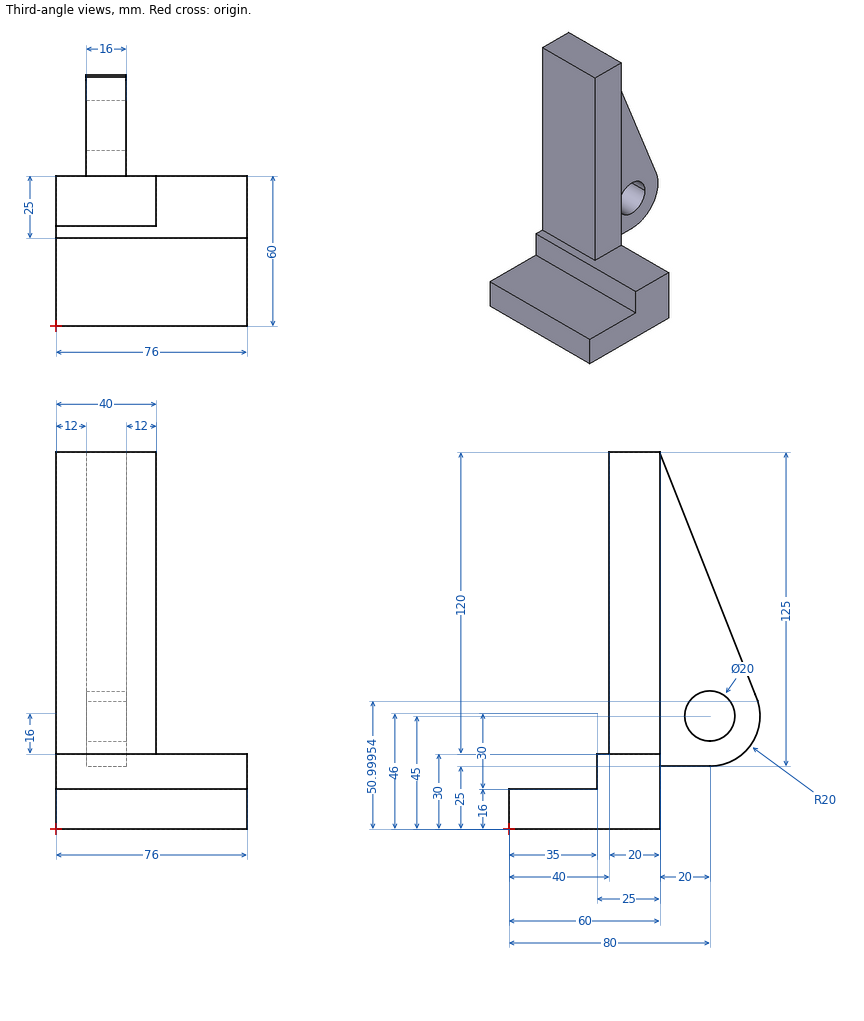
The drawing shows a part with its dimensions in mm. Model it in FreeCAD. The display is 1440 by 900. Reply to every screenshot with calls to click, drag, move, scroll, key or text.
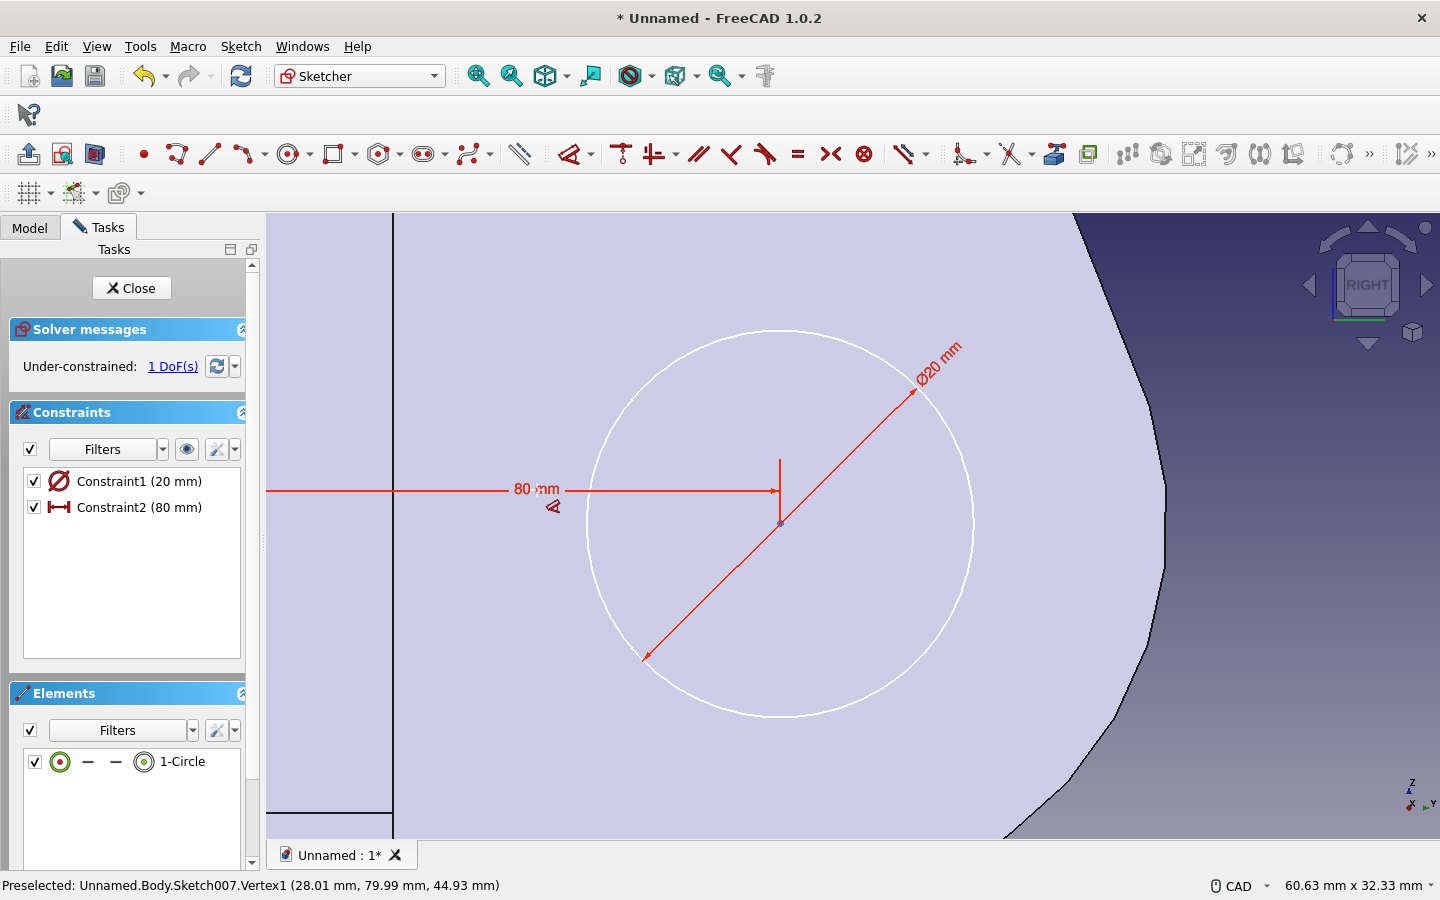
click(780, 524)
click(814, 668)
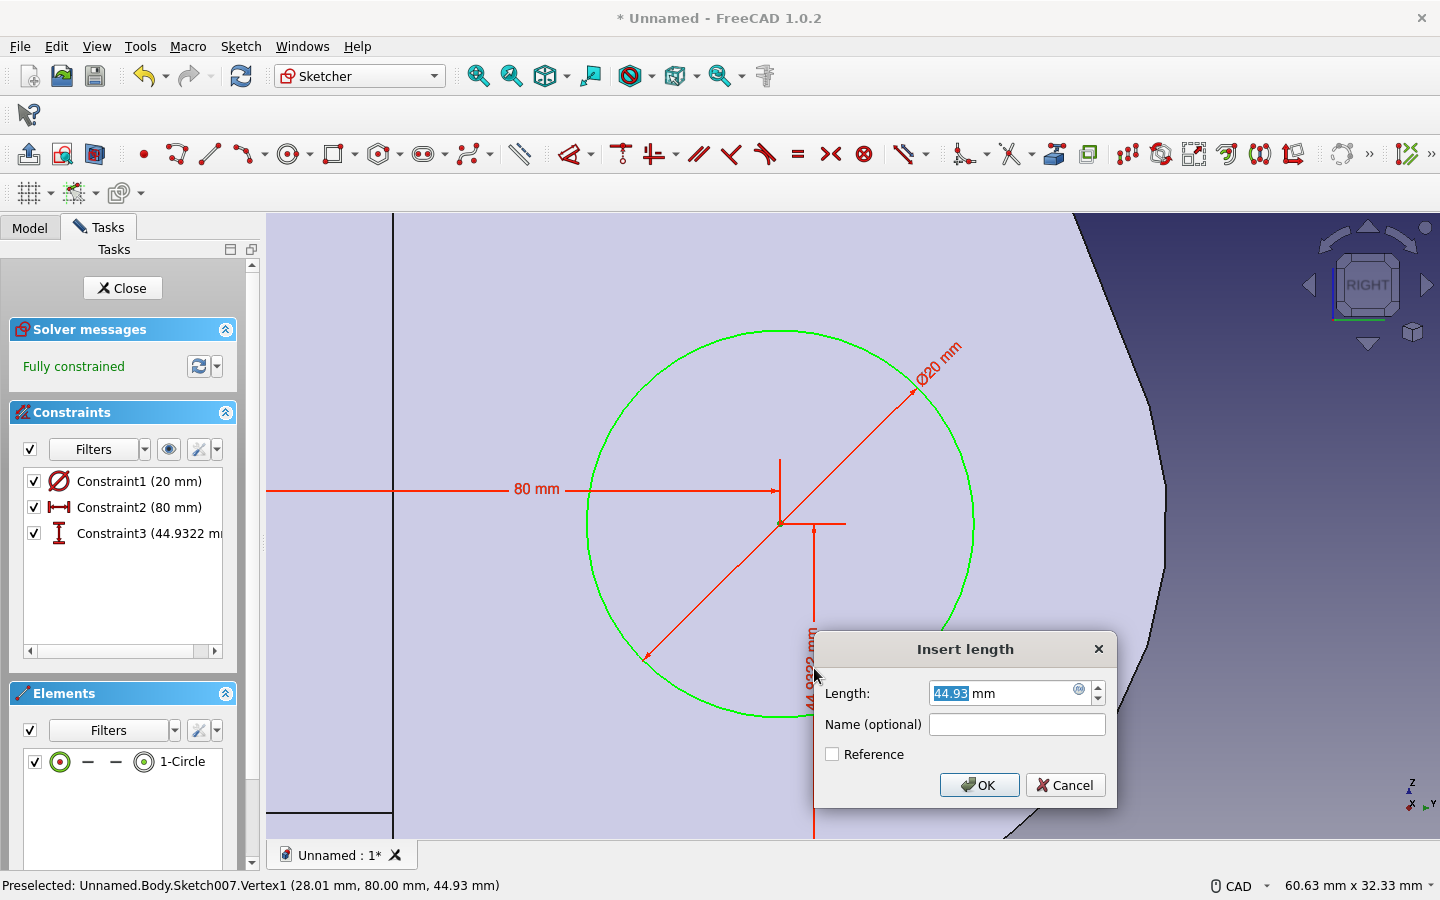
text(45)
key(Return)
key(Escape)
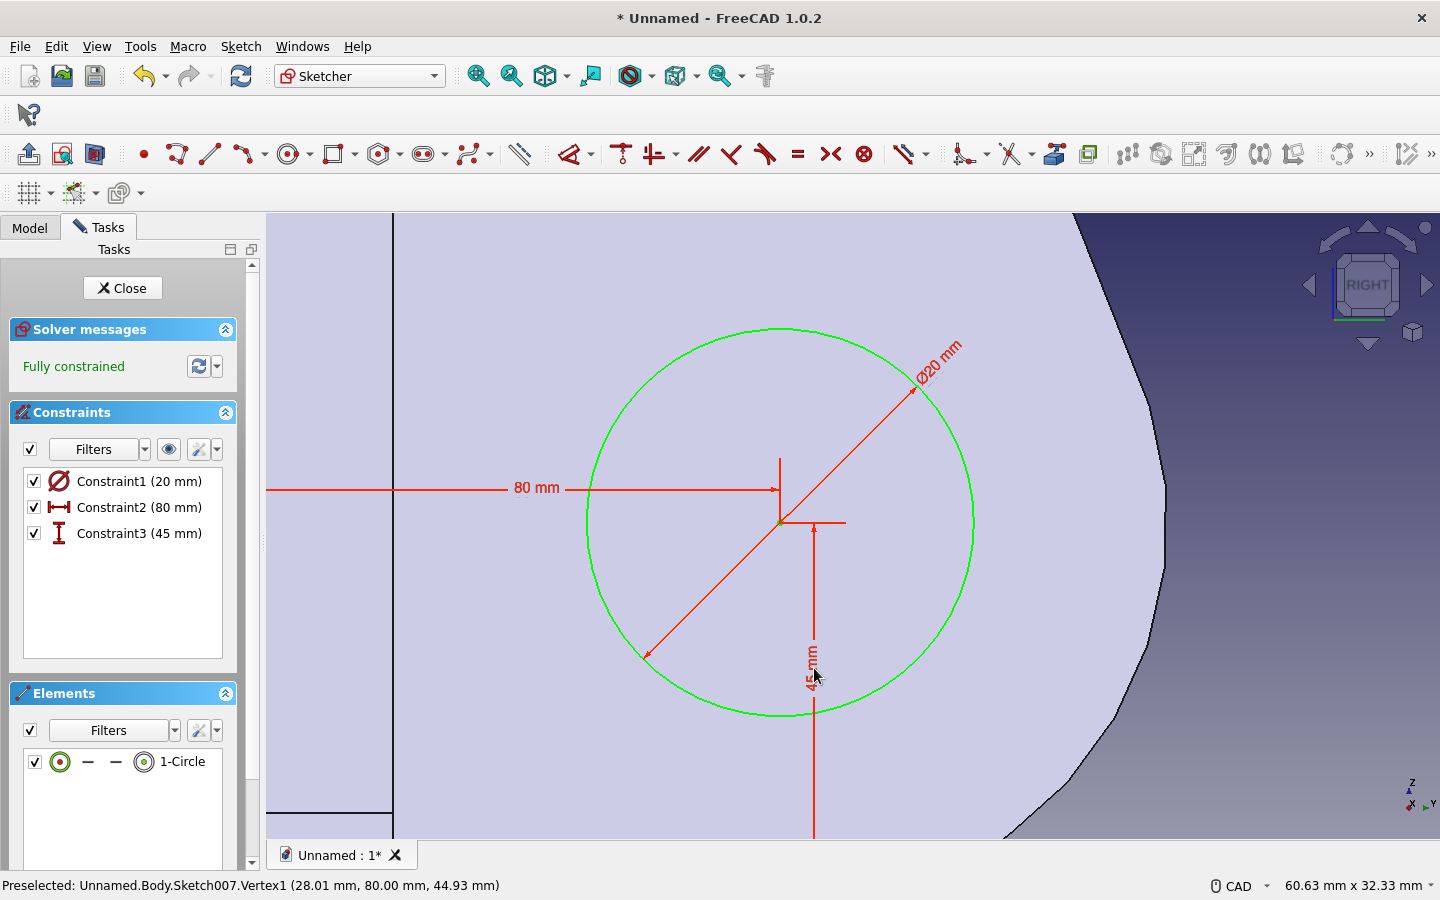
click(123, 288)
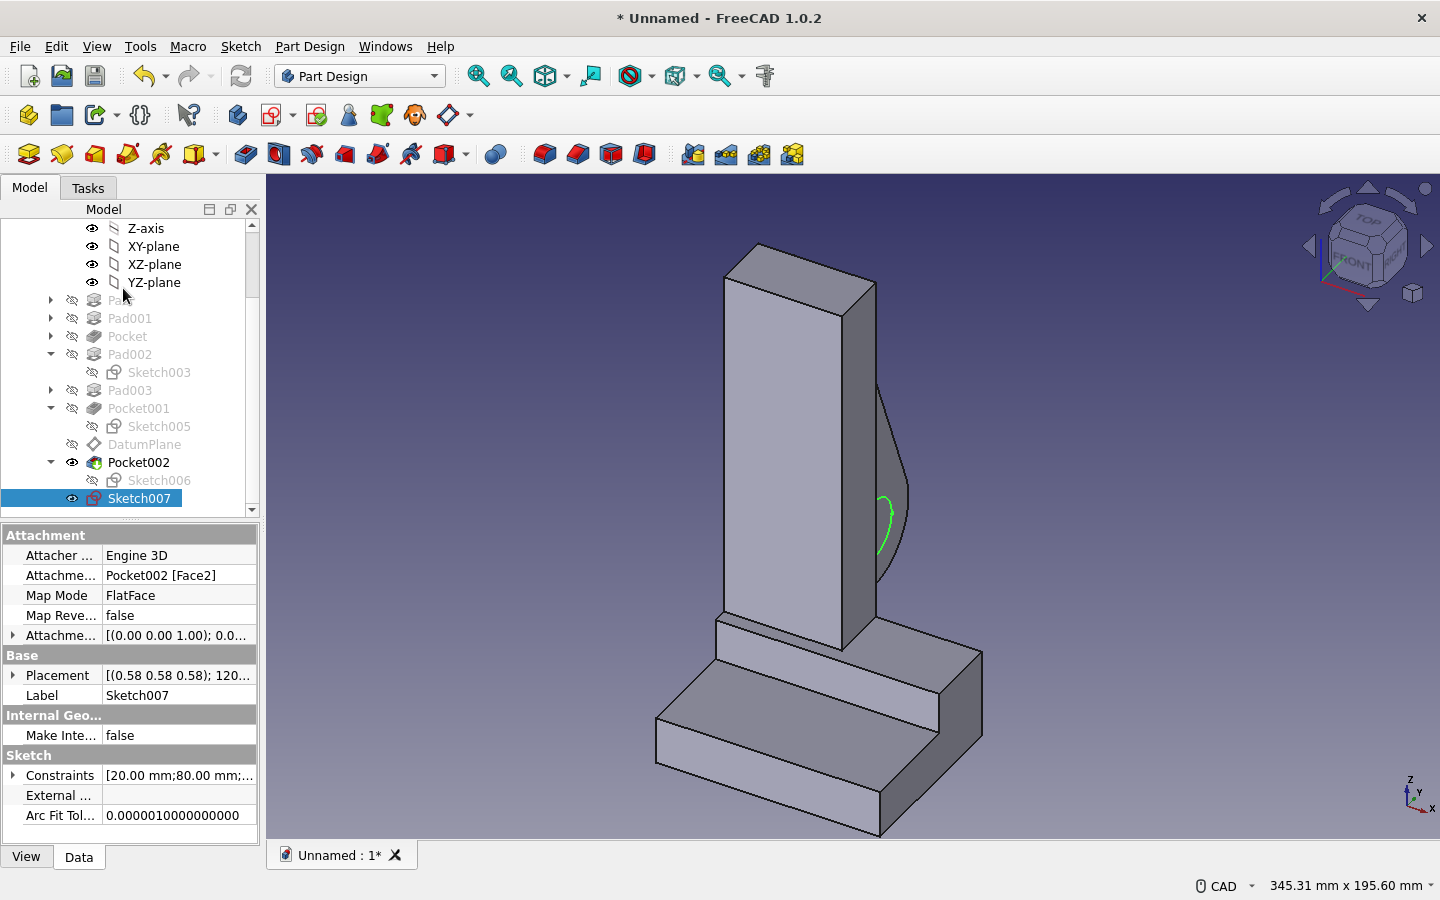
click(246, 154)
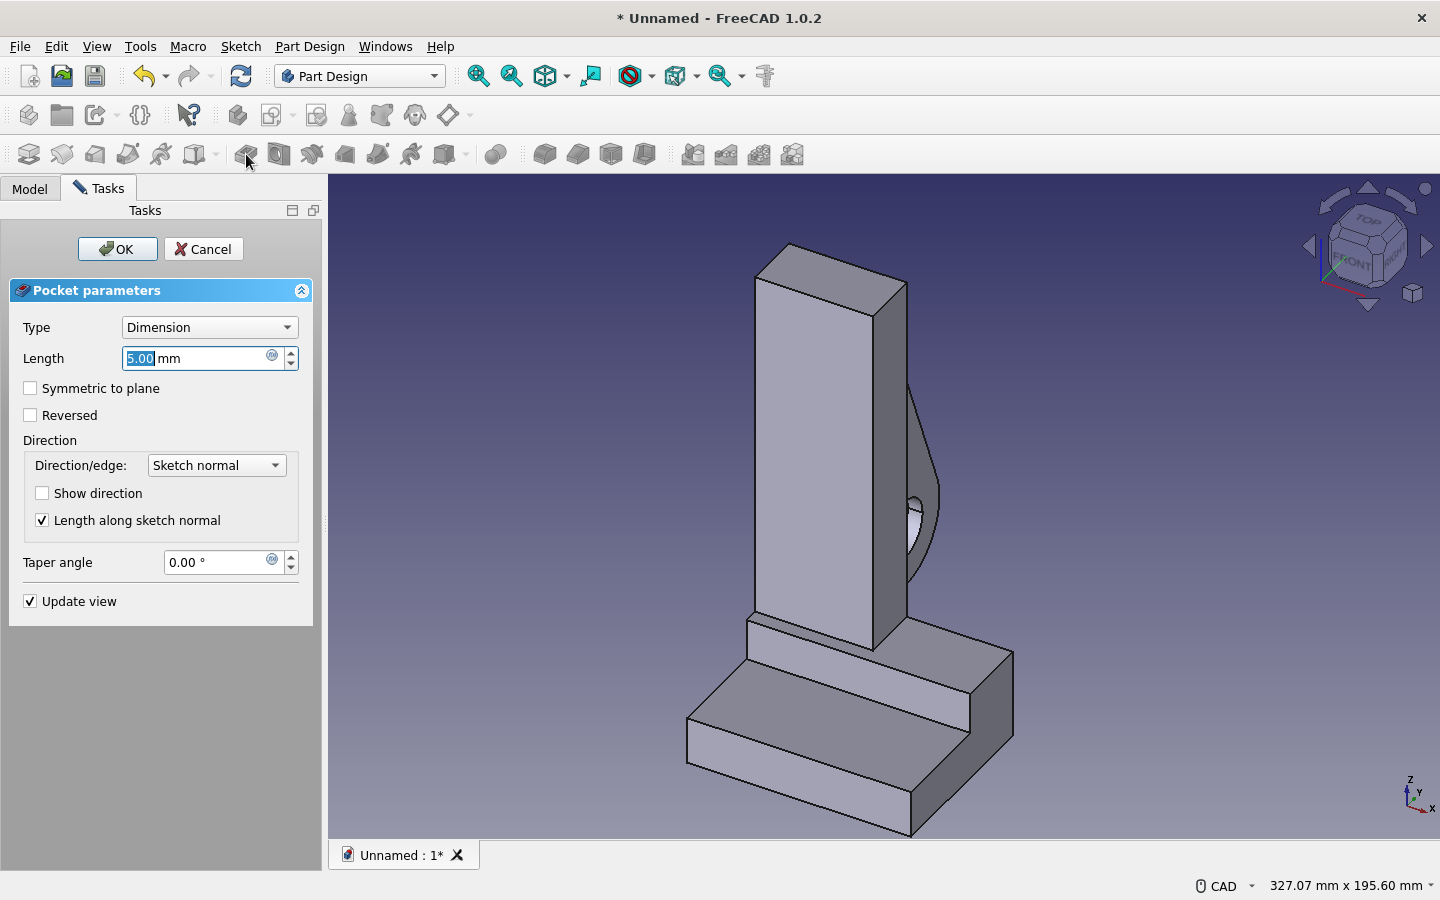
text(16)
key(Tab)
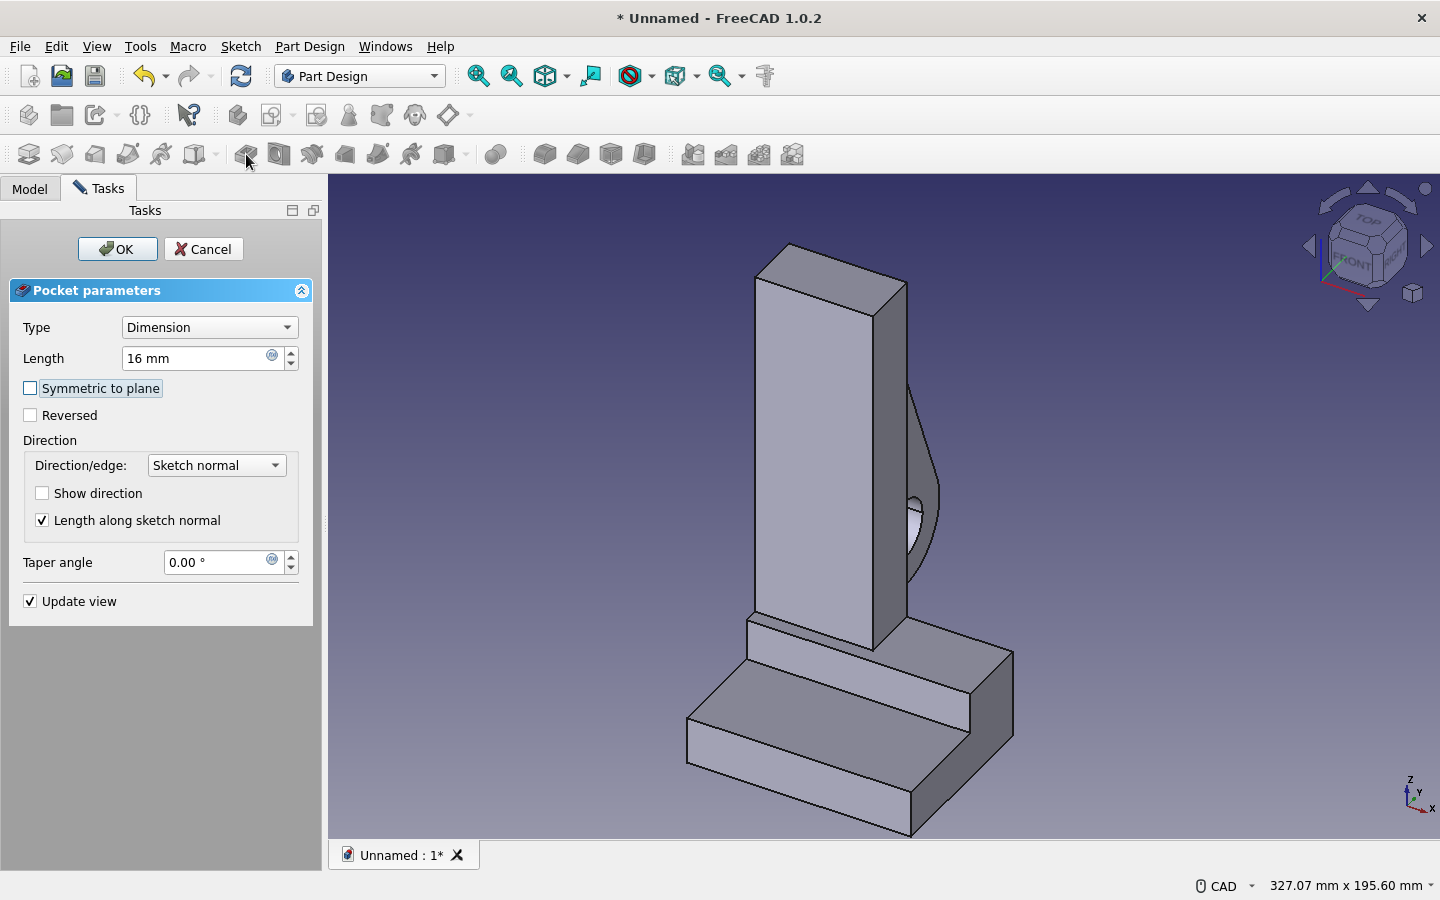
click(118, 249)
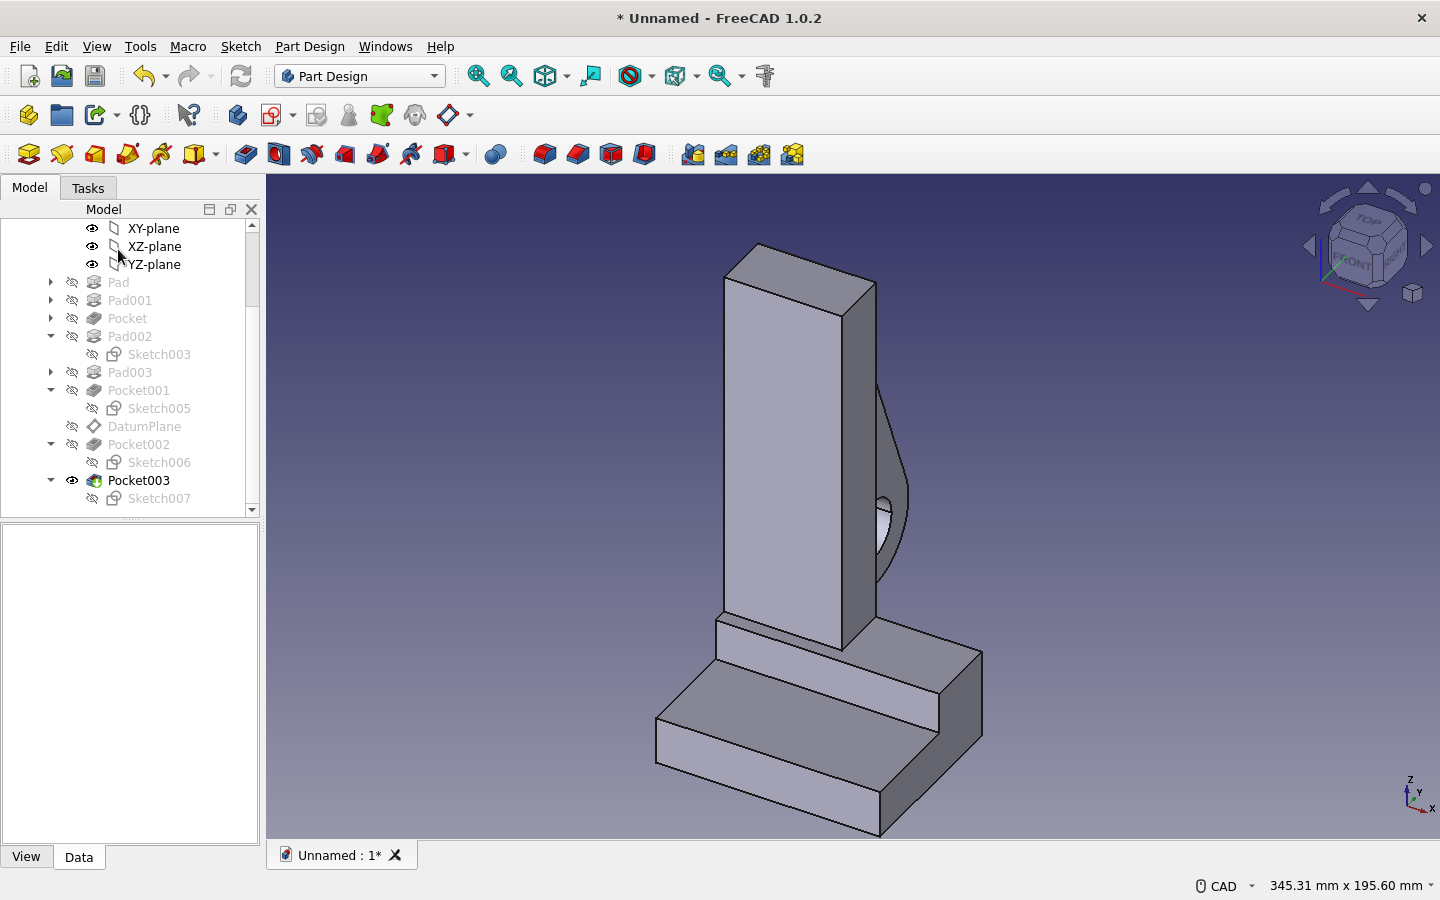
key(0)